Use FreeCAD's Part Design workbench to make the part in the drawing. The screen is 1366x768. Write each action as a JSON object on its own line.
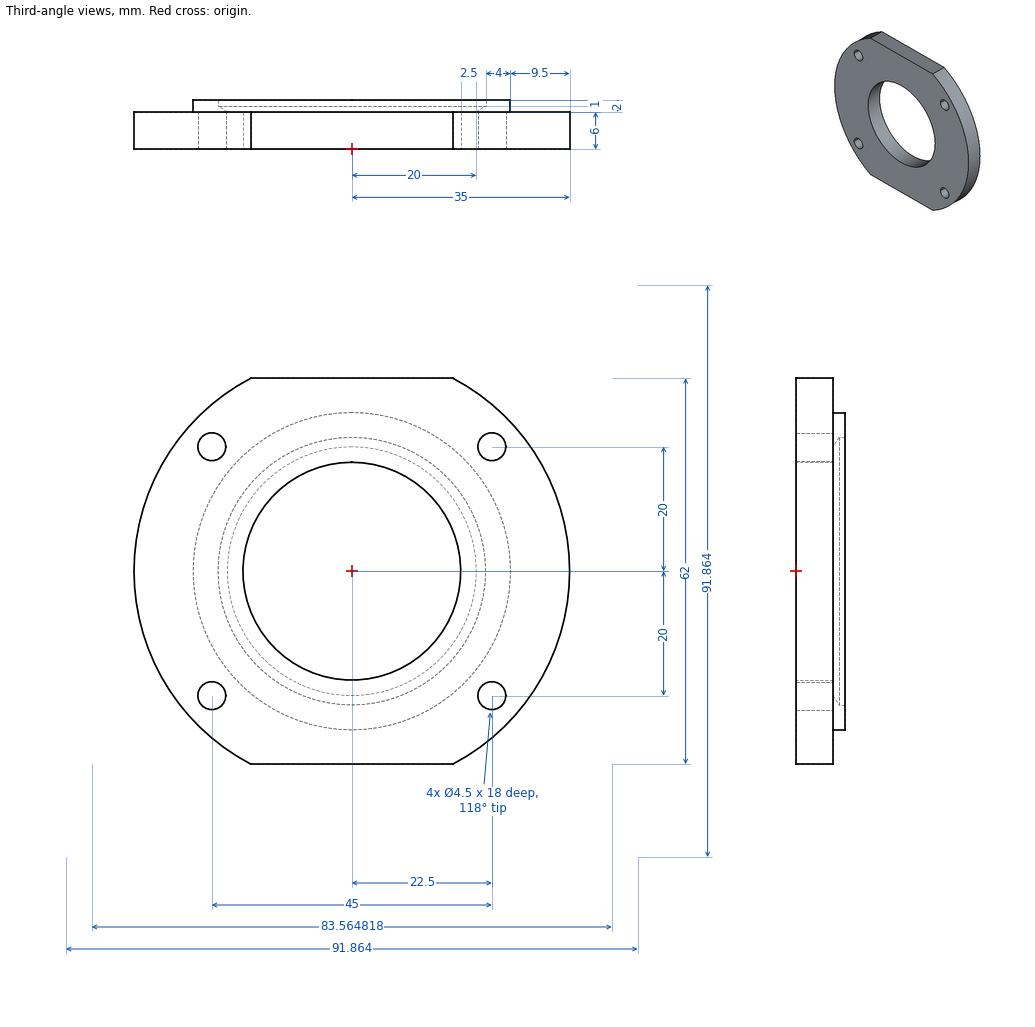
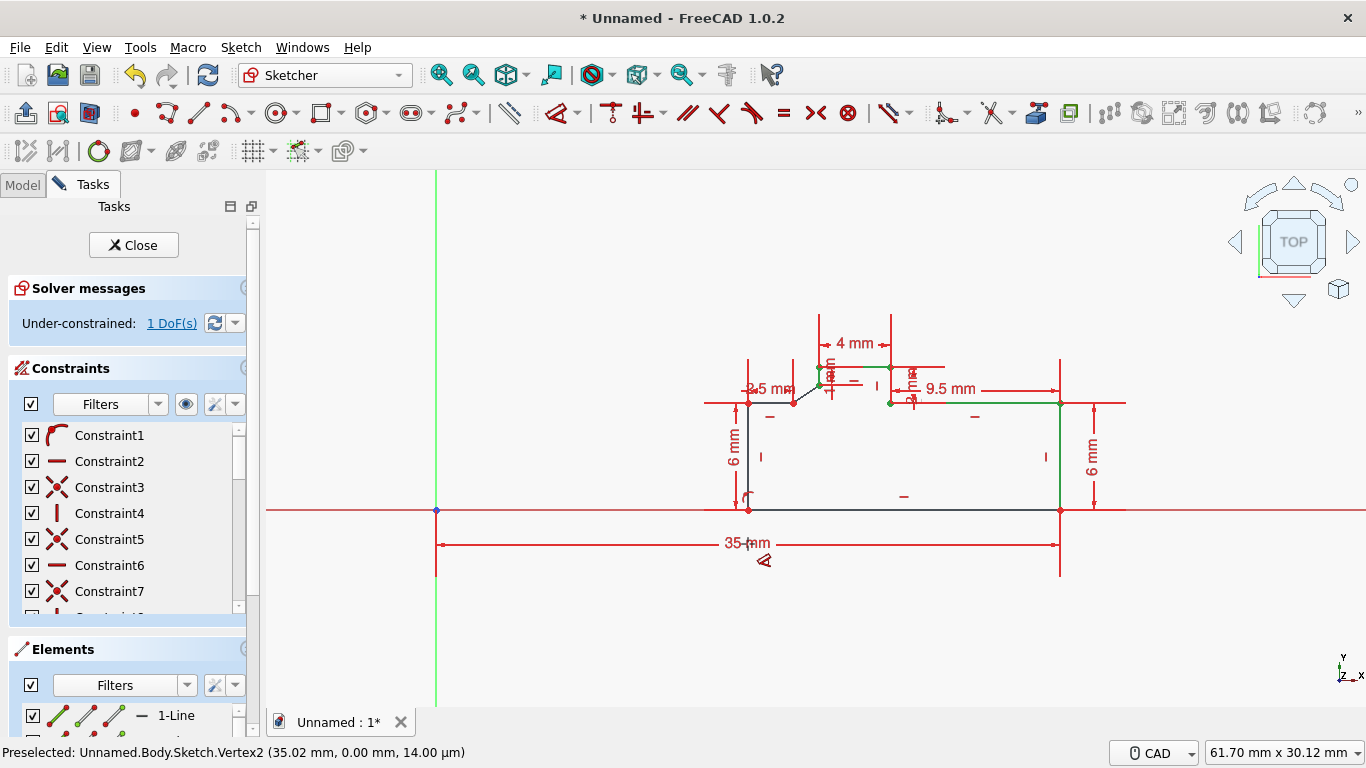
{"action": "left_click", "coordinate": [793, 403]}
{"action": "left_click", "coordinate": [615, 544]}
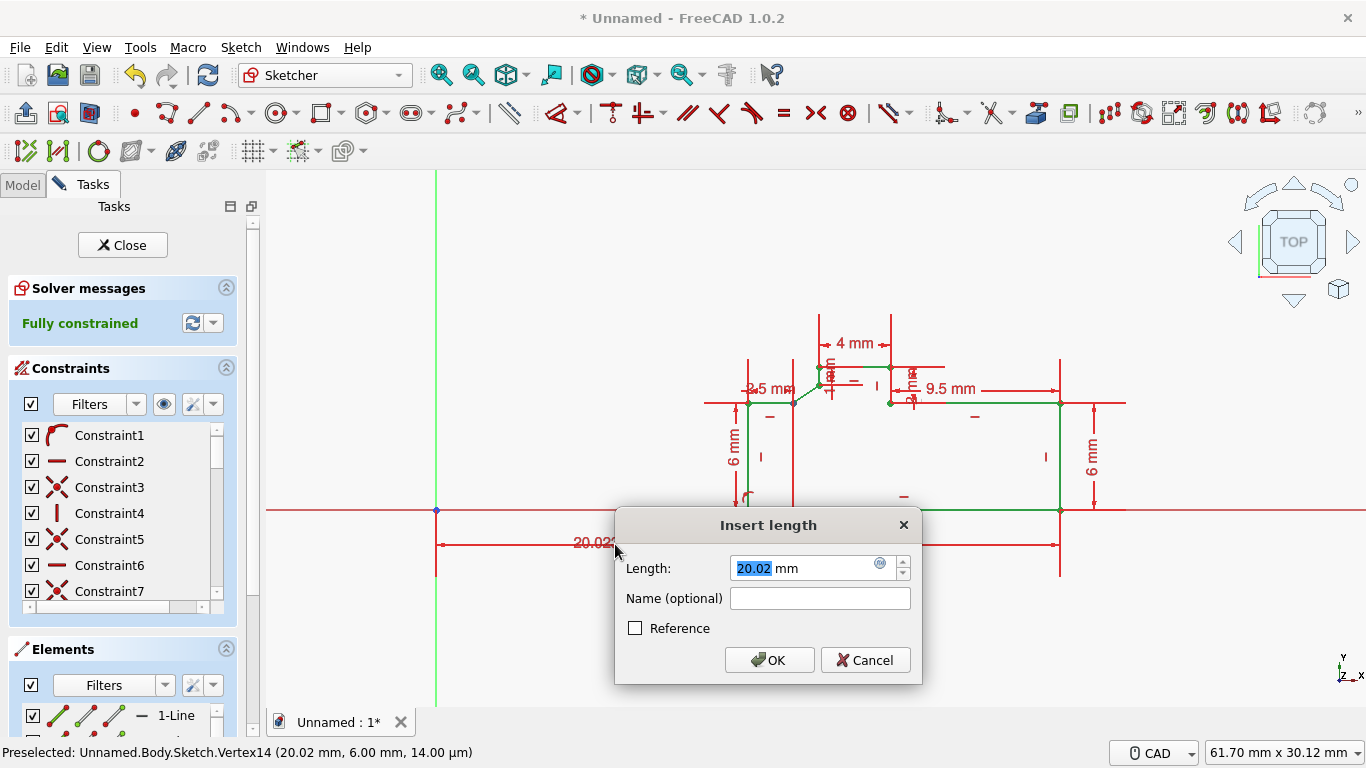
{"action": "type", "text": "20"}
{"action": "key", "text": "Return"}
{"action": "key", "text": "Escape"}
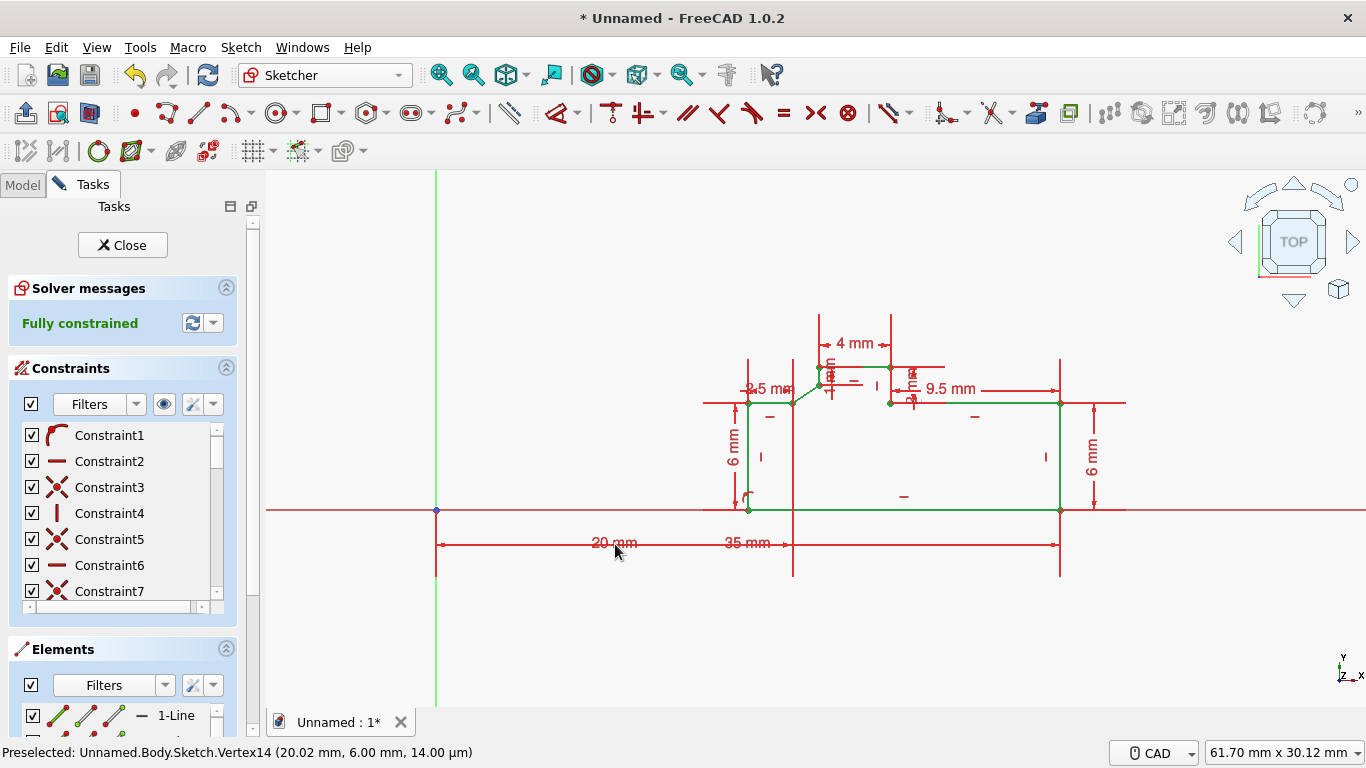
{"action": "left_click", "coordinate": [123, 245]}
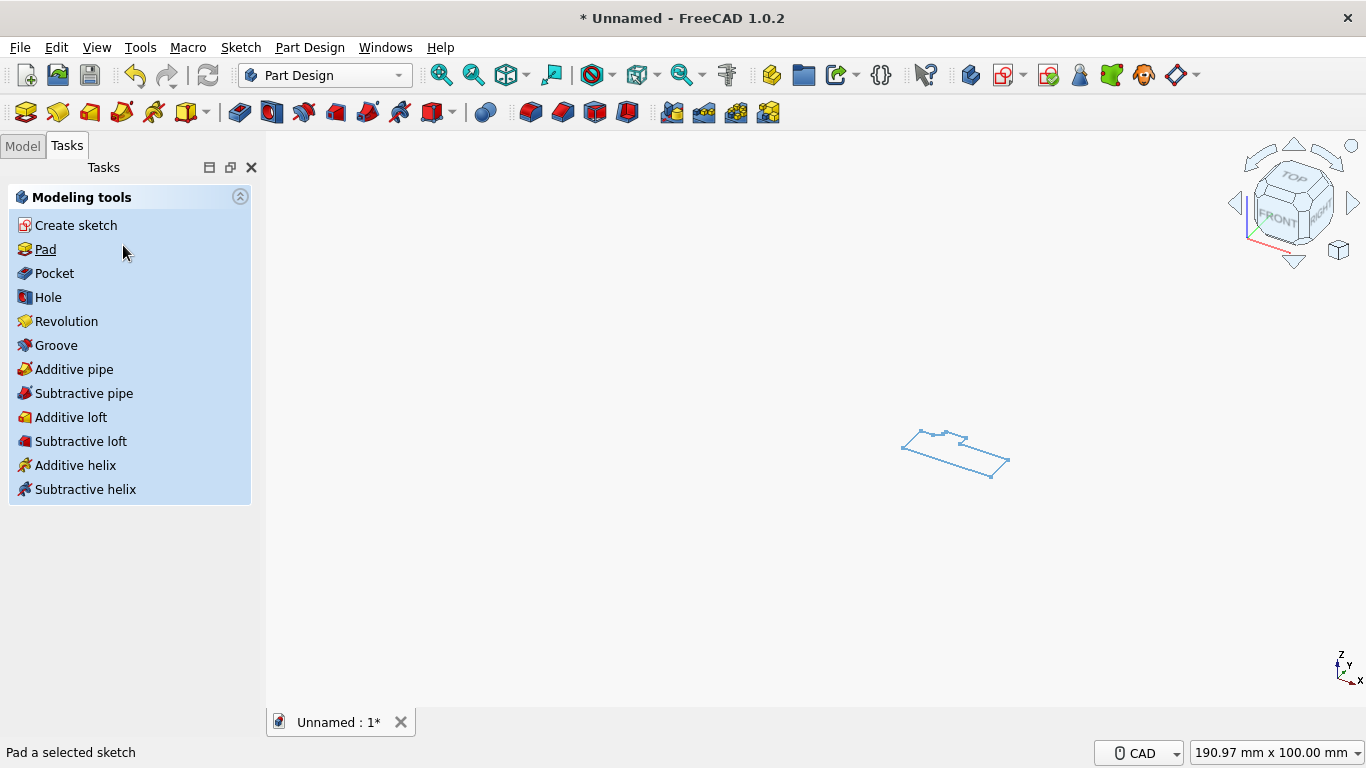
{"action": "left_click", "coordinate": [58, 112]}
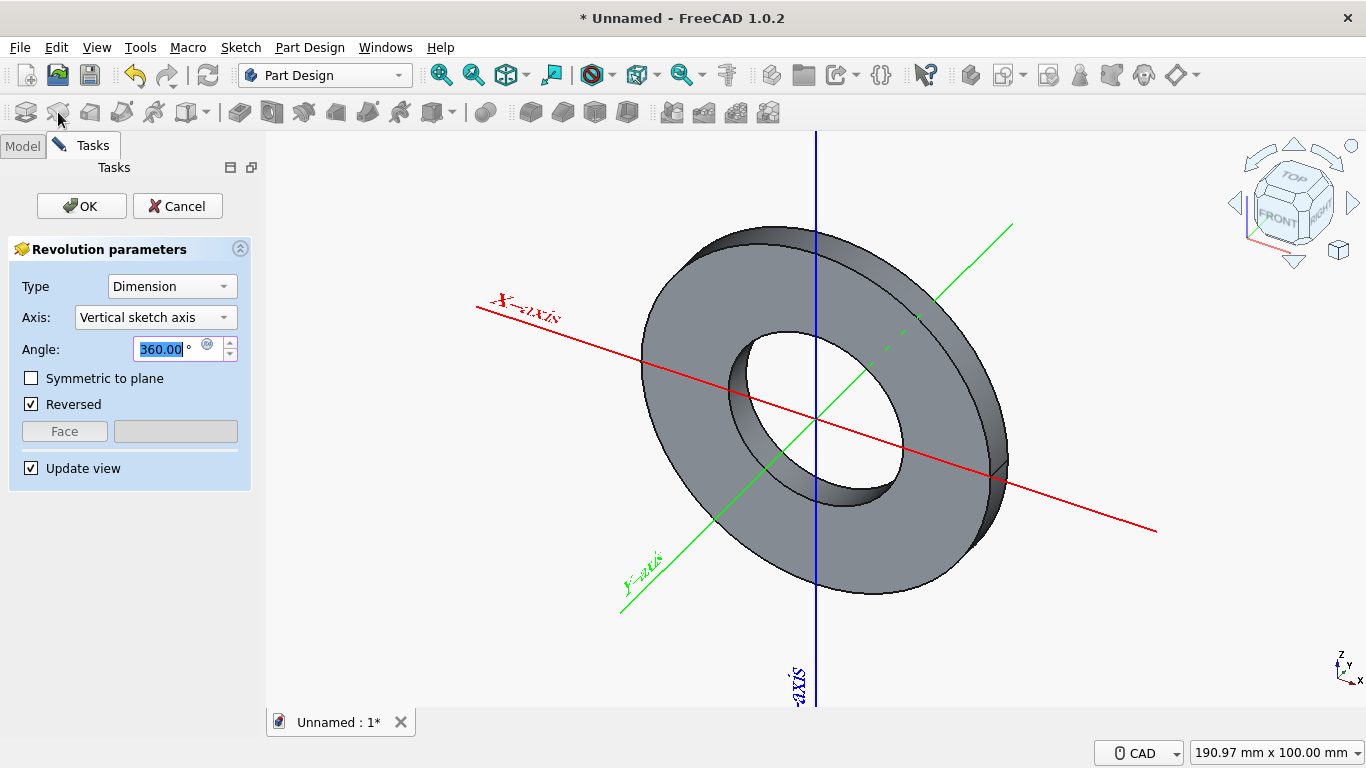
{"action": "left_click", "coordinate": [82, 206]}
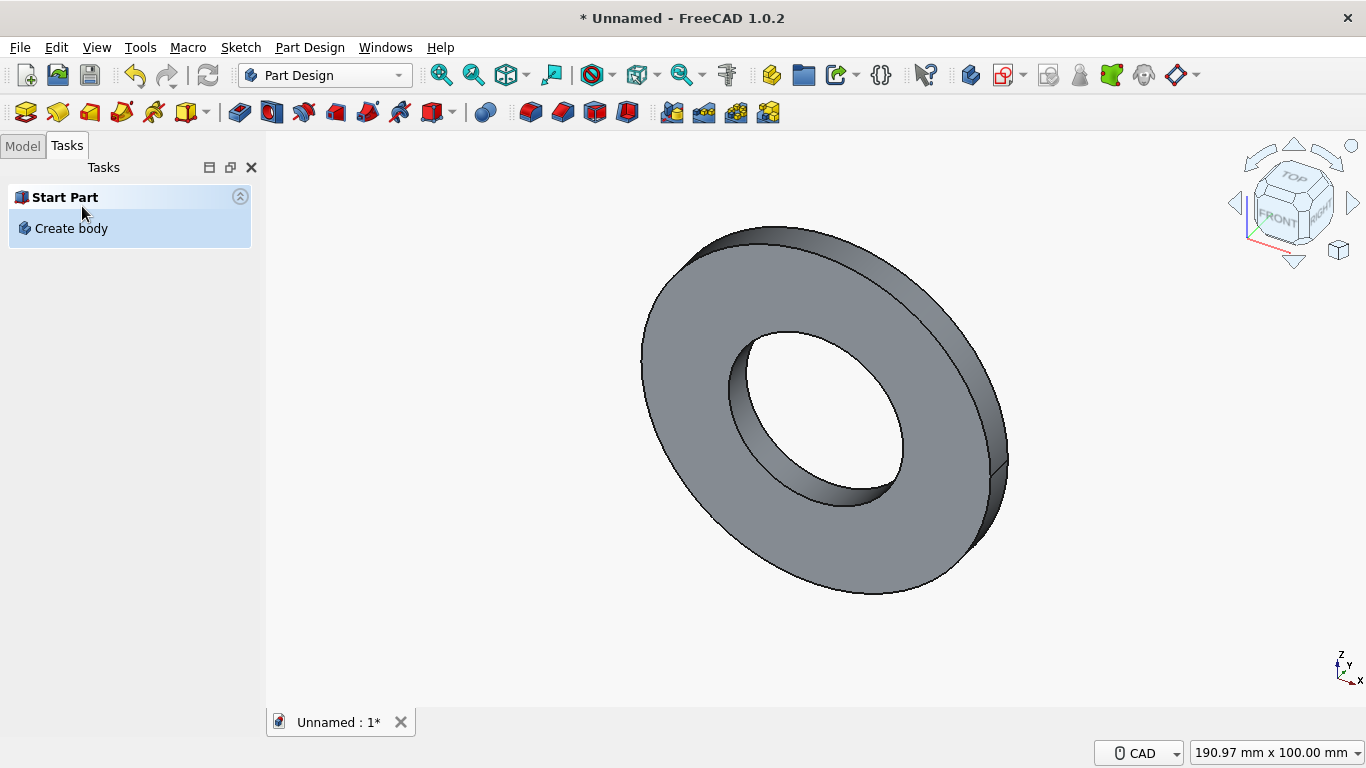
{"action": "left_click", "coordinate": [716, 479]}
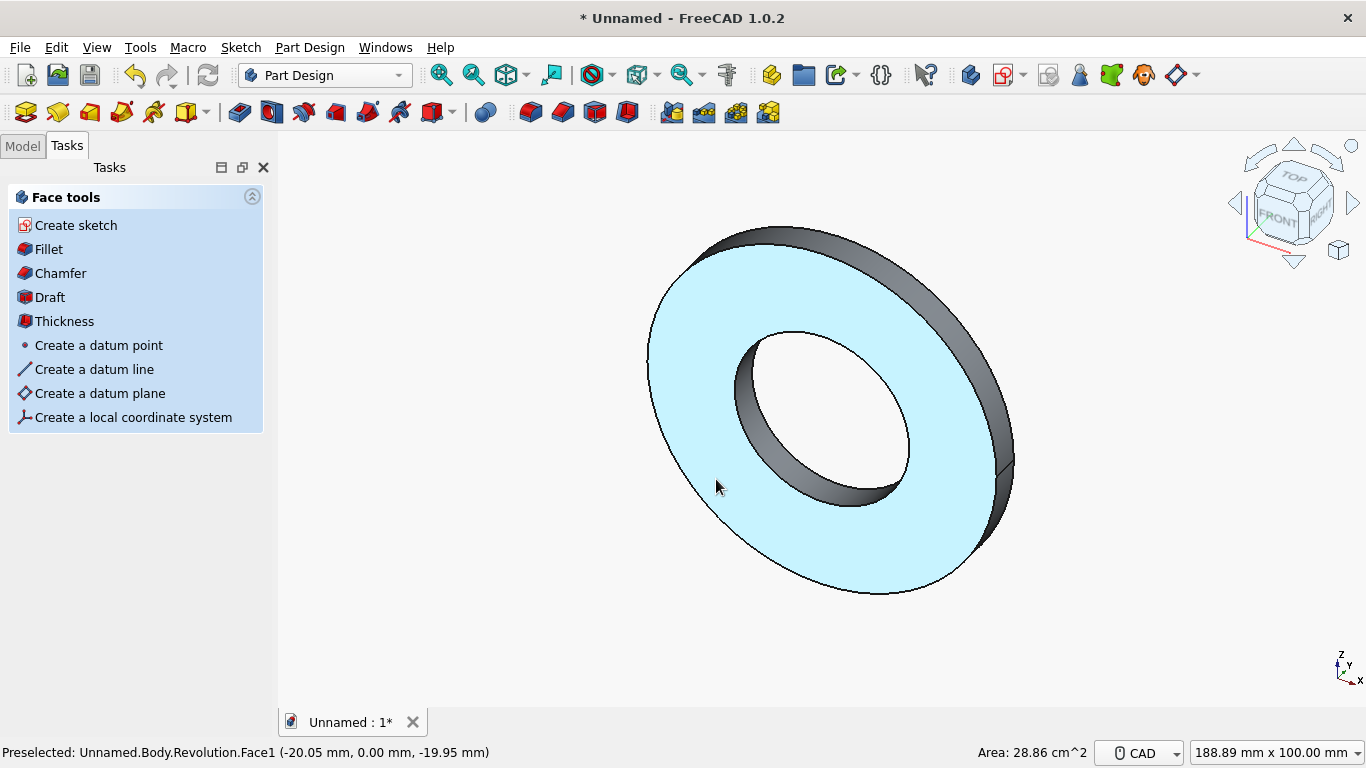
{"action": "left_click", "coordinate": [1004, 76]}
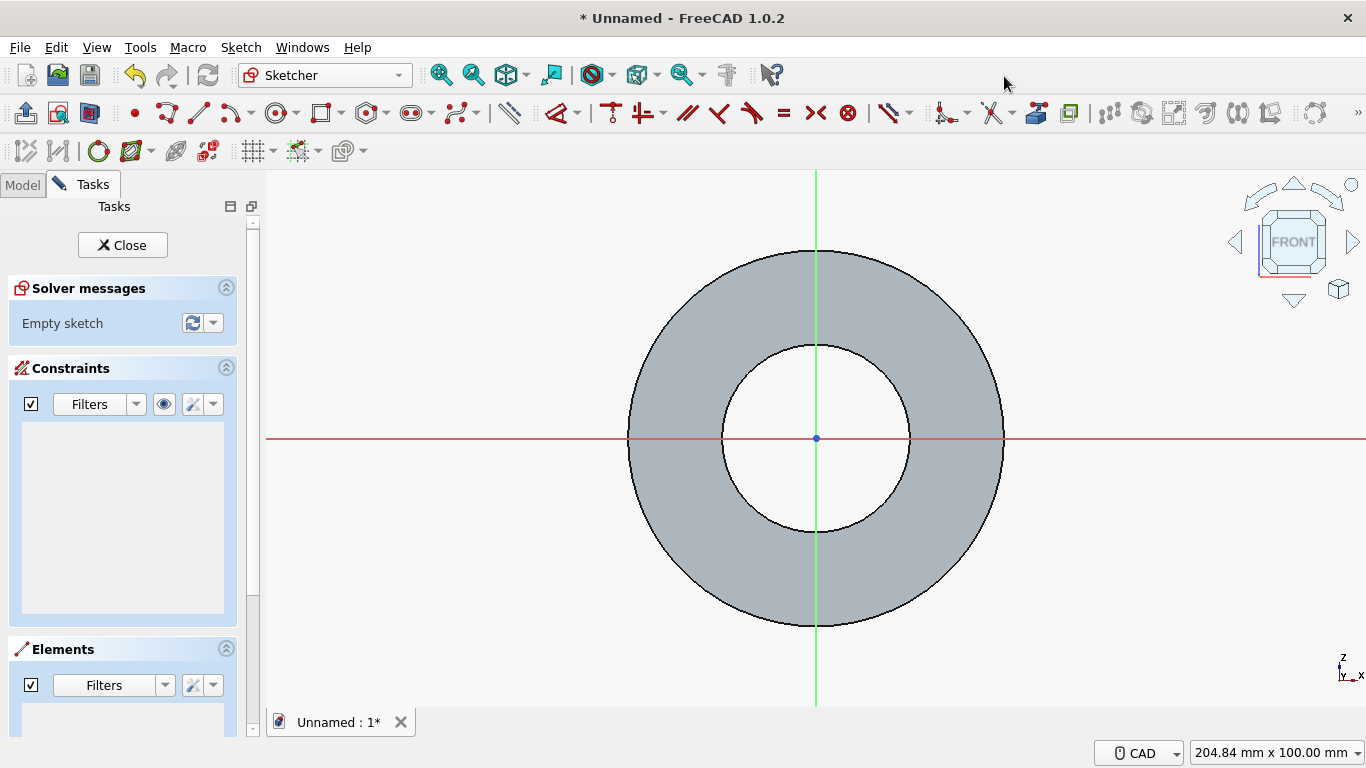
{"action": "scroll", "coordinate": [955, 438], "scroll_direction": "up", "scroll_amount": 2}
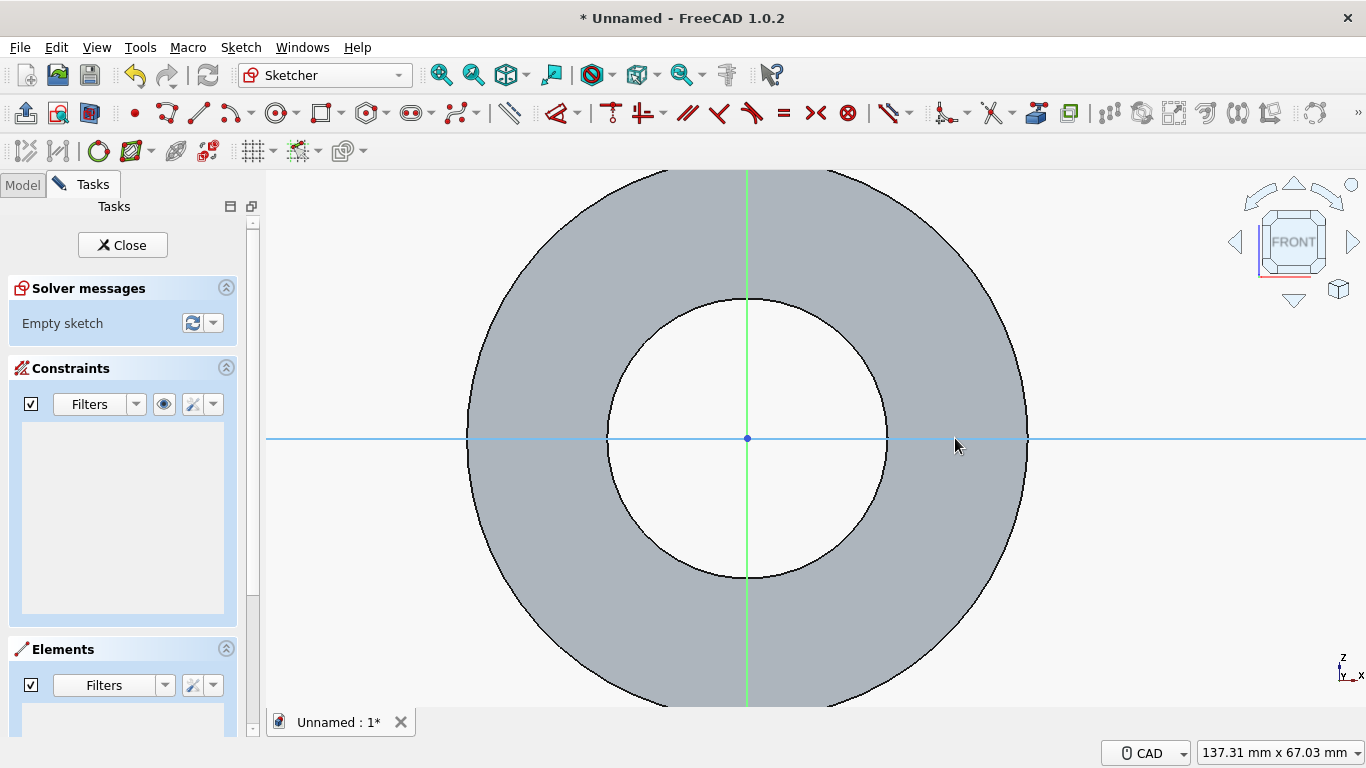
{"action": "left_click", "coordinate": [276, 114]}